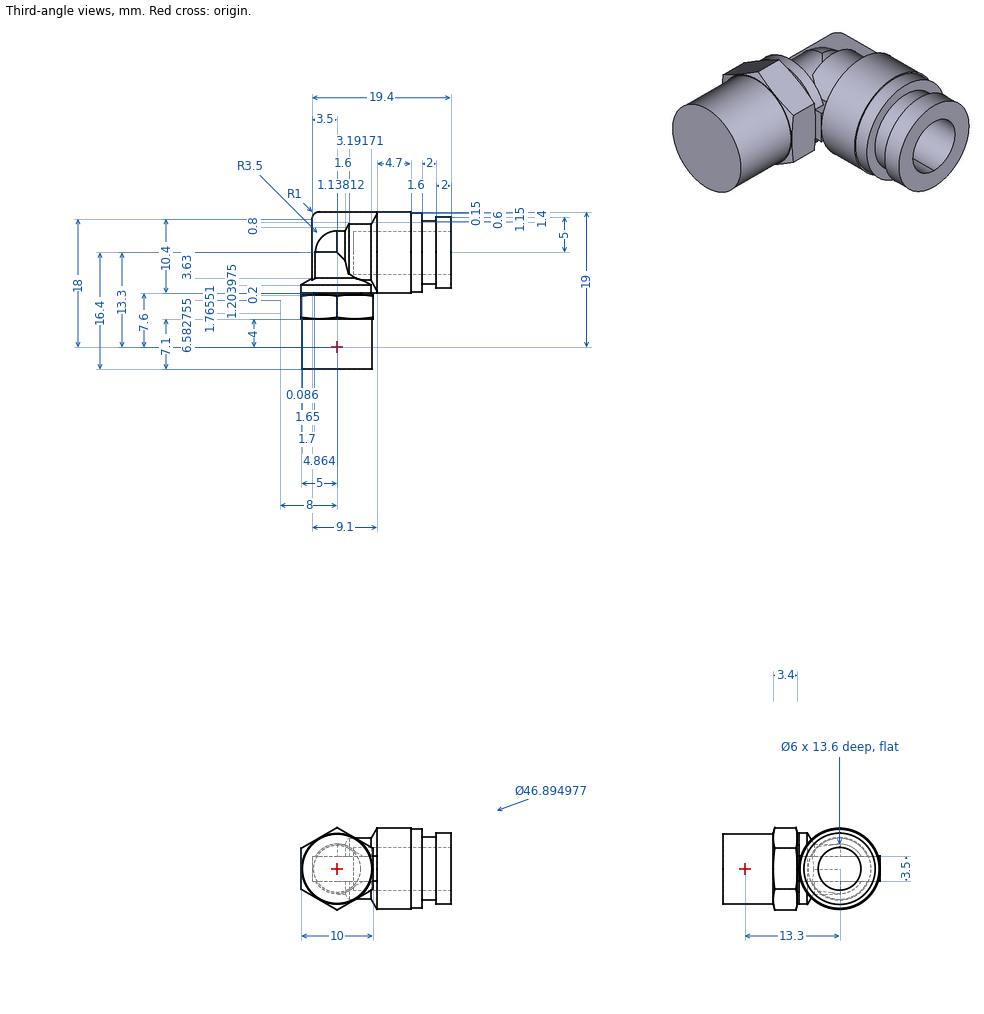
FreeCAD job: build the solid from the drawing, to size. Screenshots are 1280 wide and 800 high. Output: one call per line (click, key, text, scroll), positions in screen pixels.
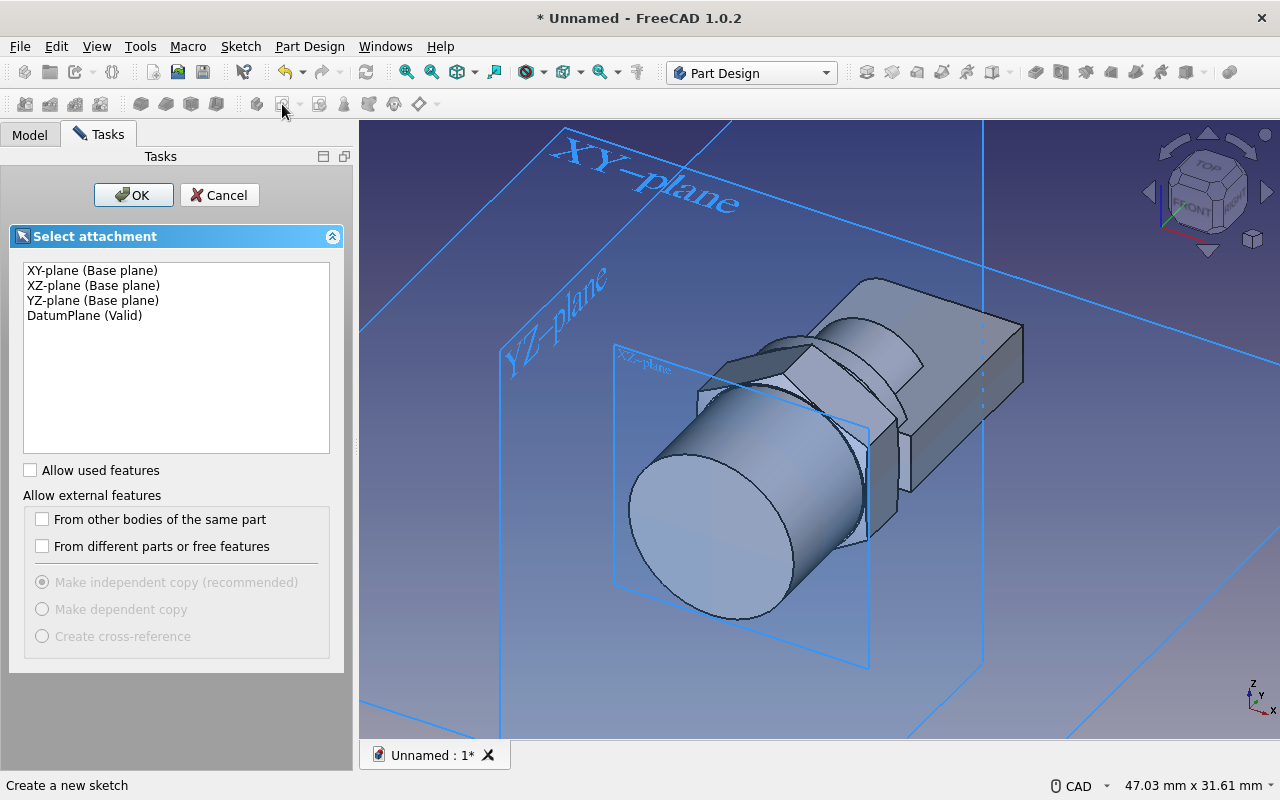
click(84, 270)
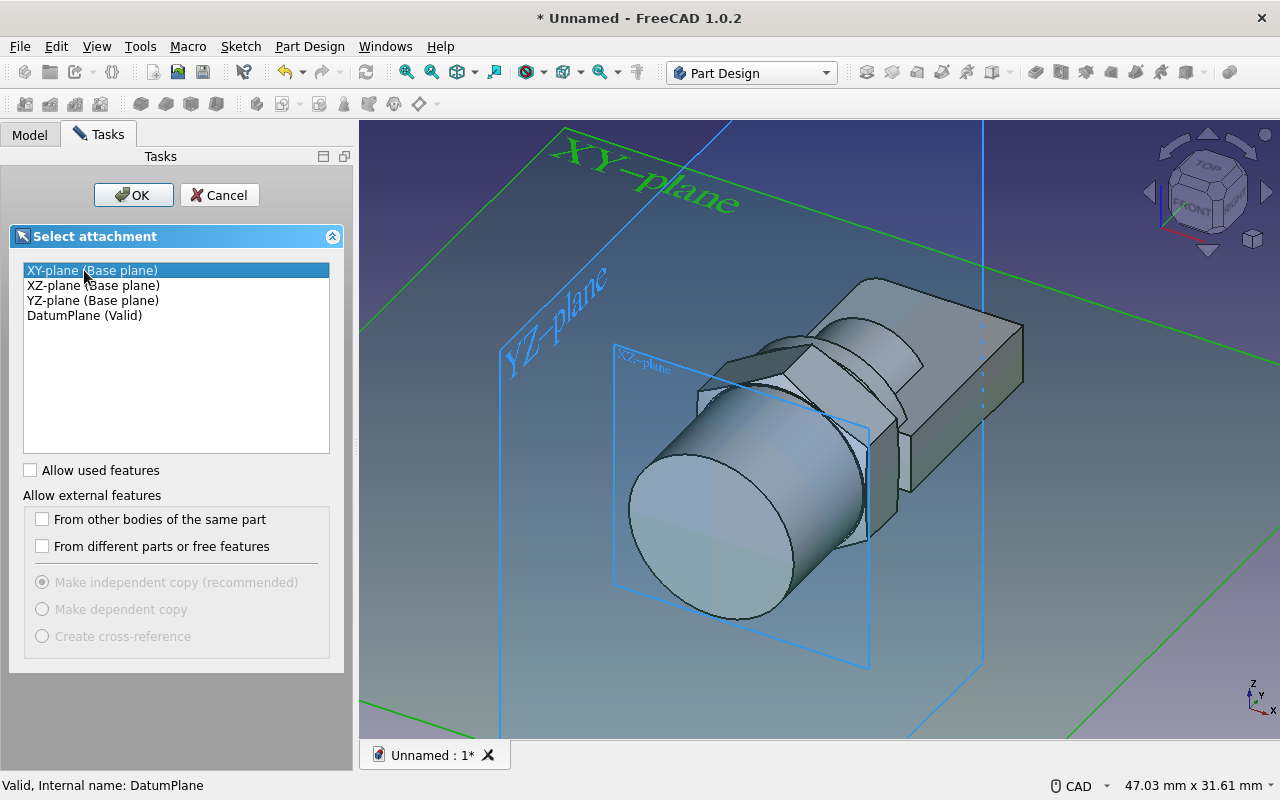
click(134, 195)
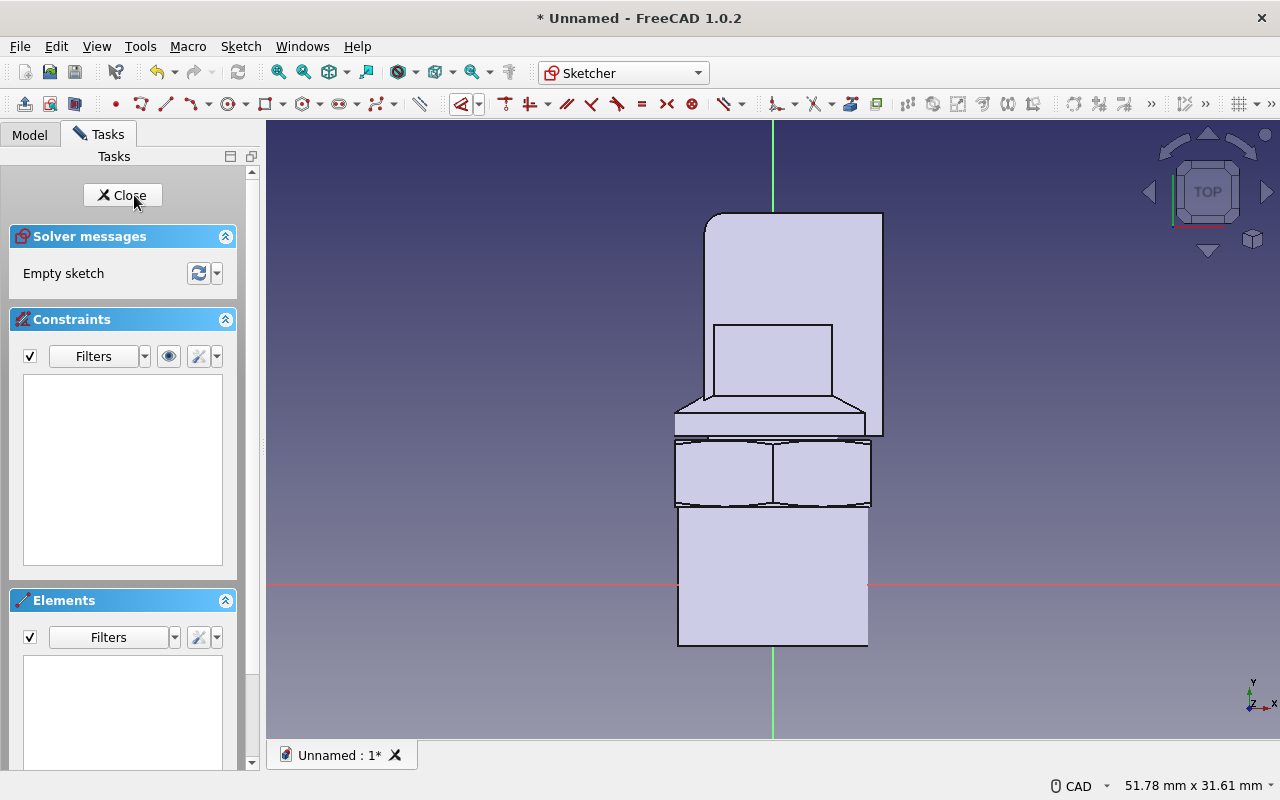
key(q)
key(s)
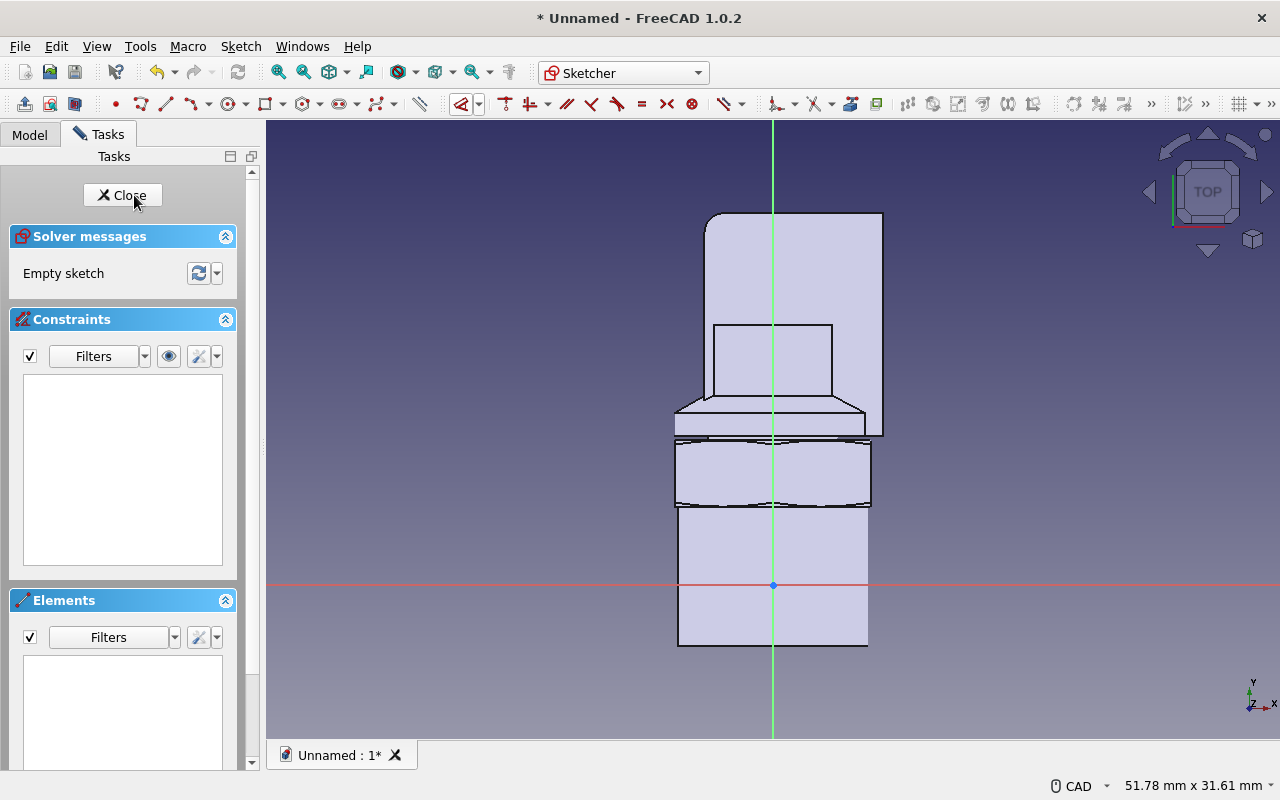
click(141, 104)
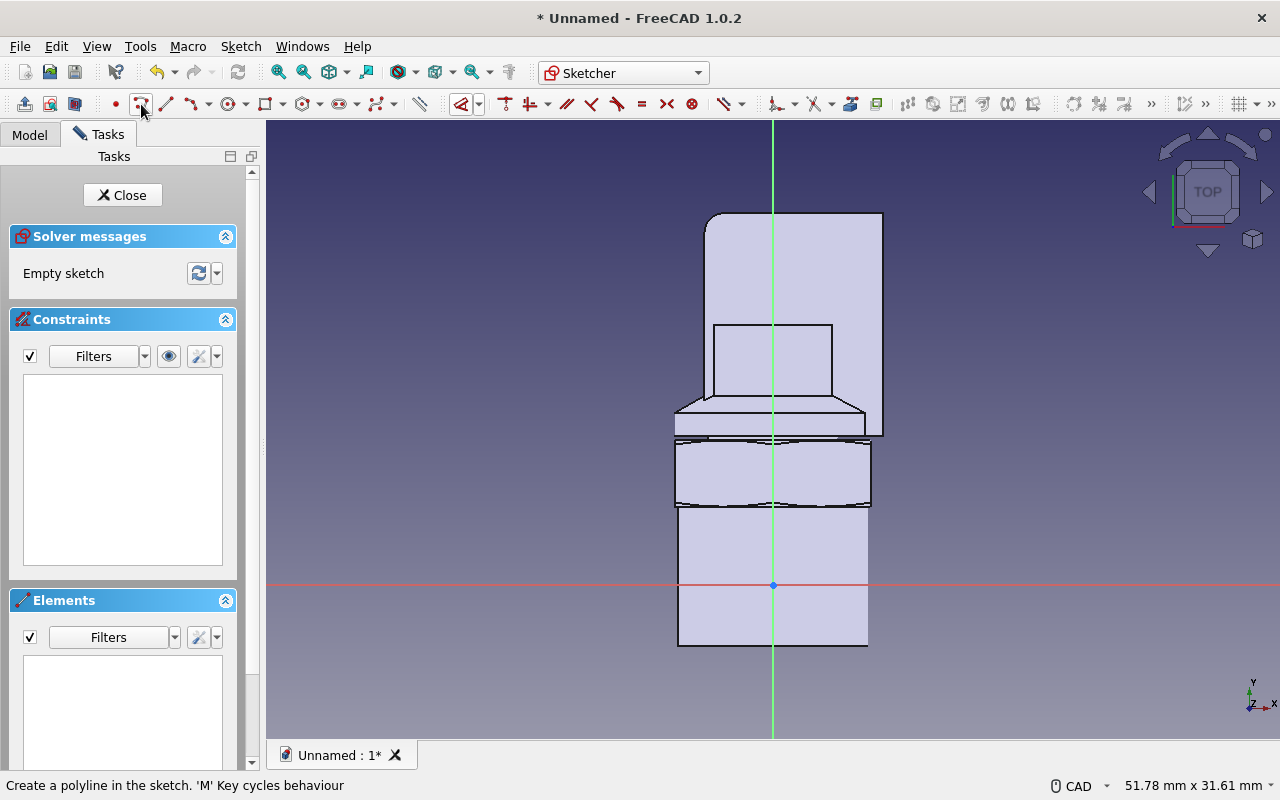
click(704, 325)
click(1084, 325)
click(1084, 227)
click(1045, 227)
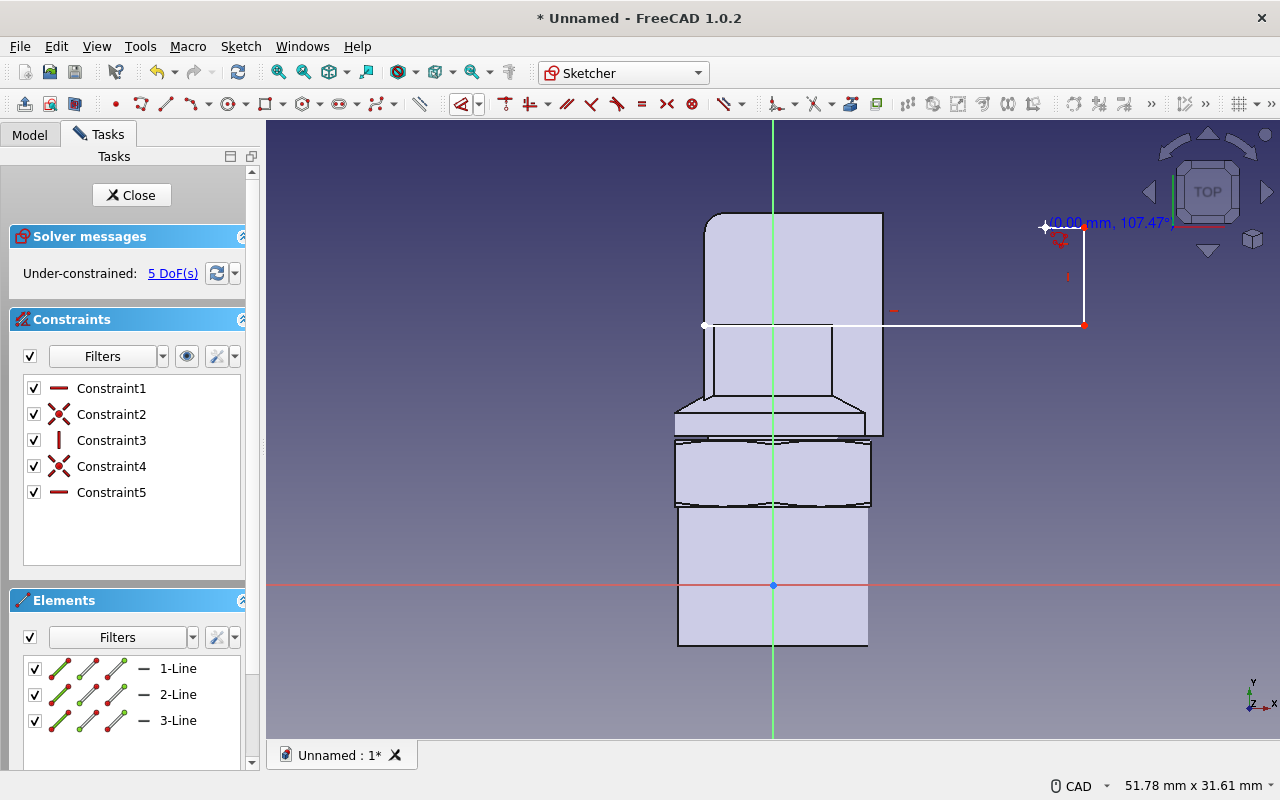
scroll(1045, 239, up, 2)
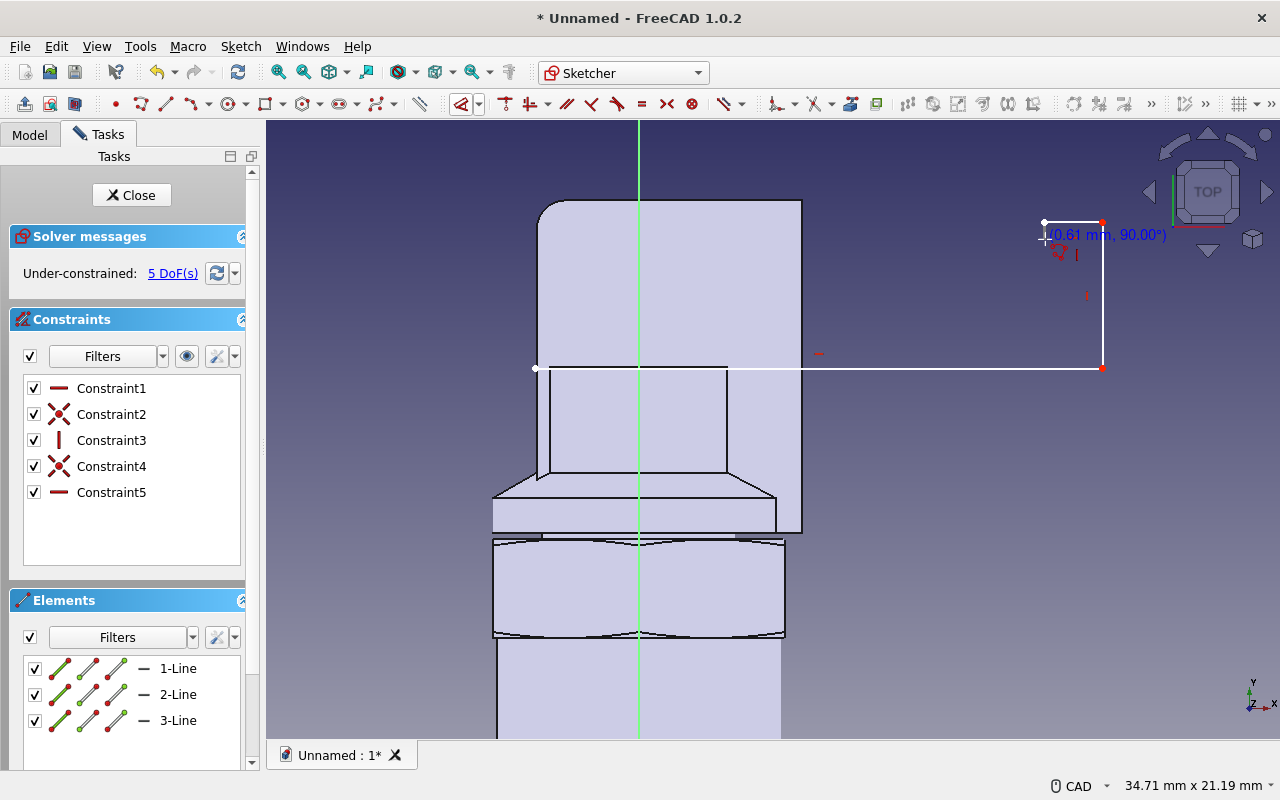
click(1045, 238)
click(986, 238)
click(986, 205)
click(940, 205)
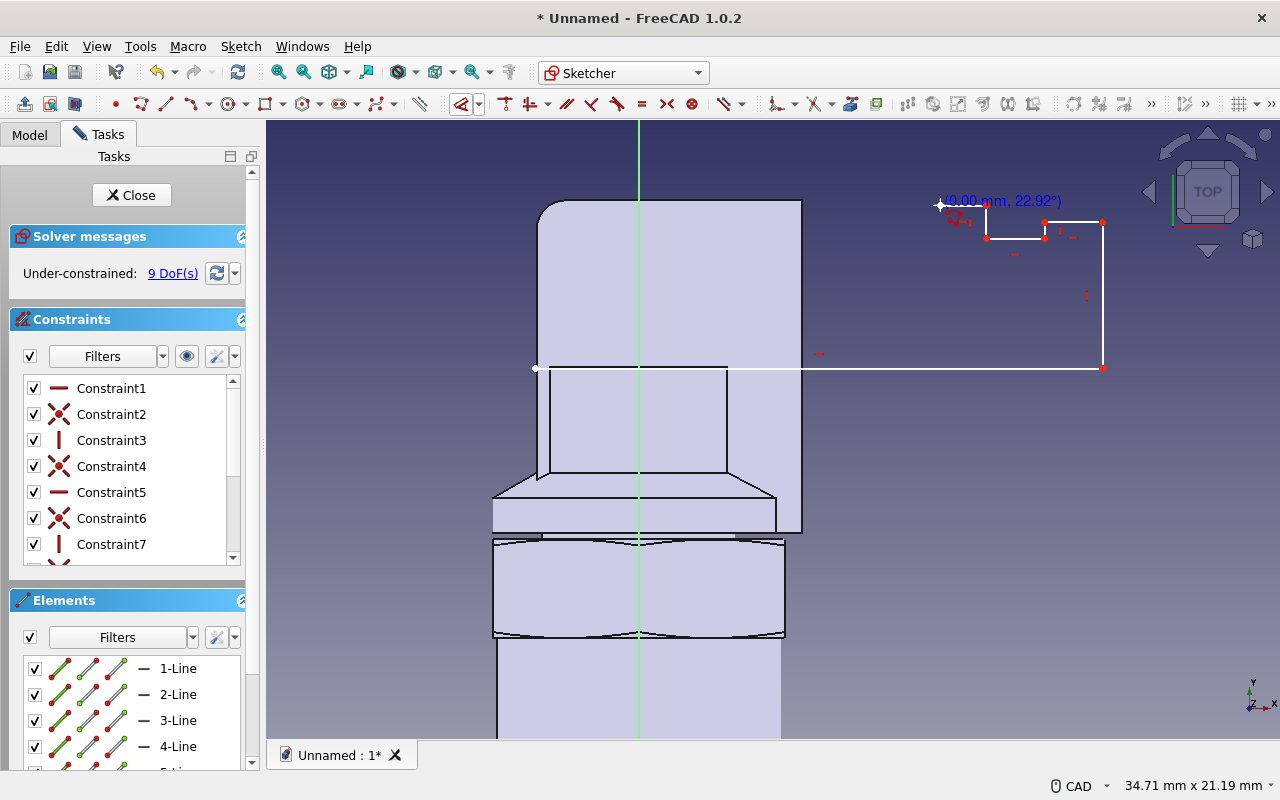
scroll(940, 200, up, 7)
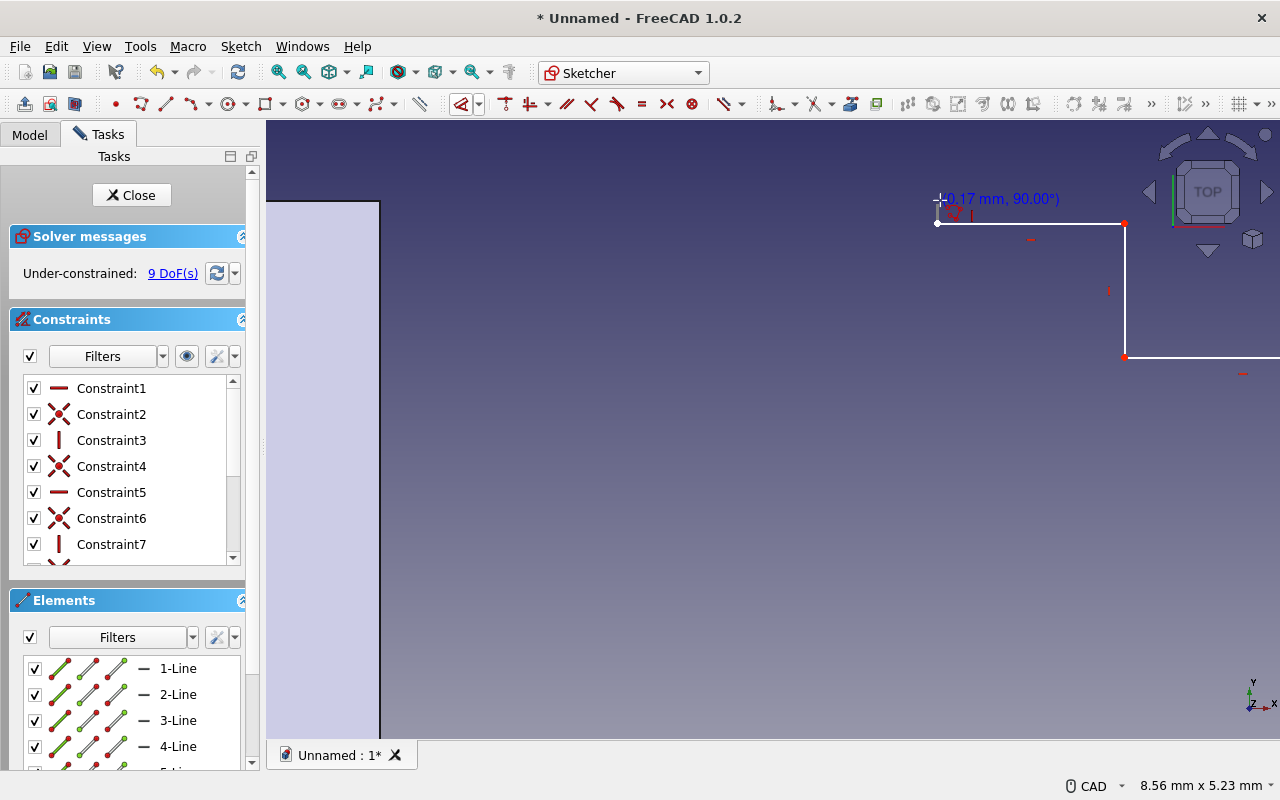
click(938, 201)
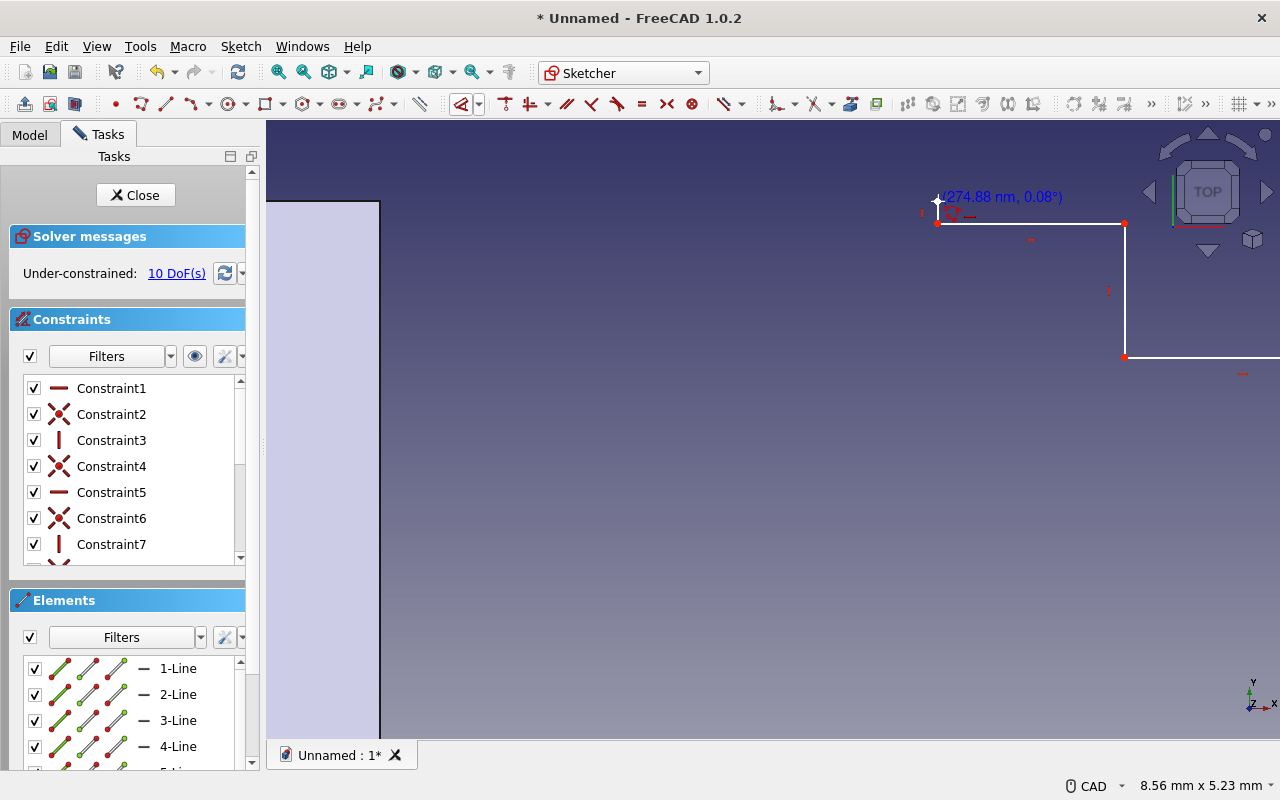
scroll(846, 252, down, 9)